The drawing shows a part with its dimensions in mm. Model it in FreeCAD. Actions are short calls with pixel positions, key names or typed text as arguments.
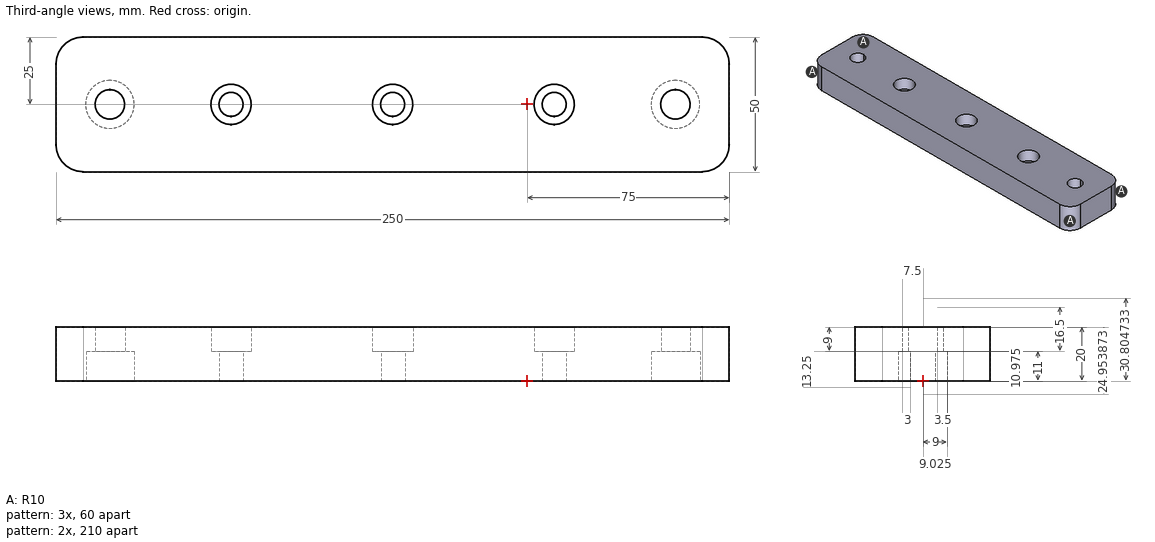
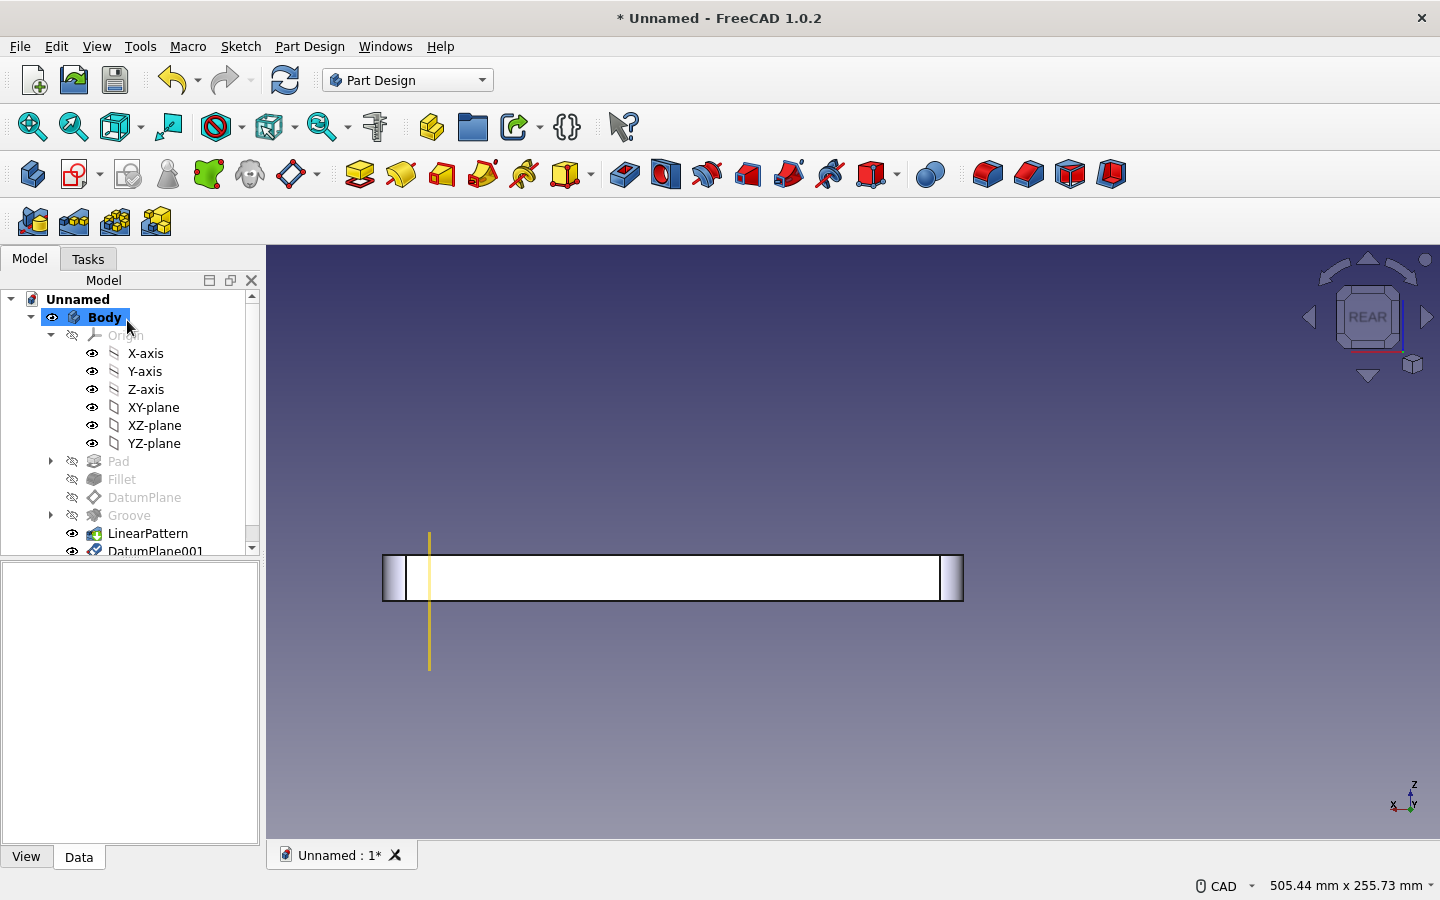
click(117, 551)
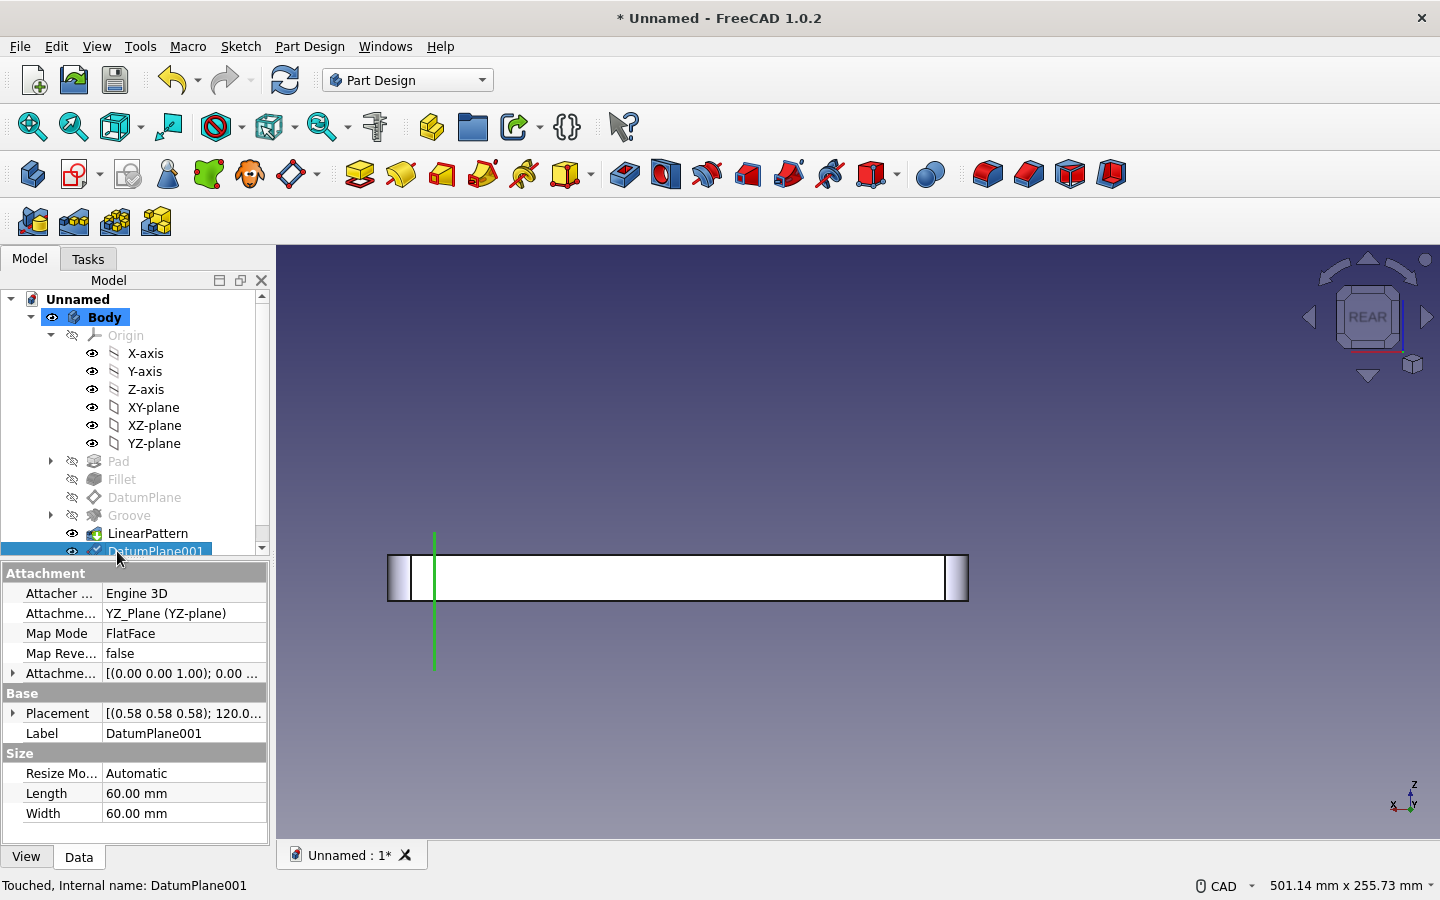
click(74, 174)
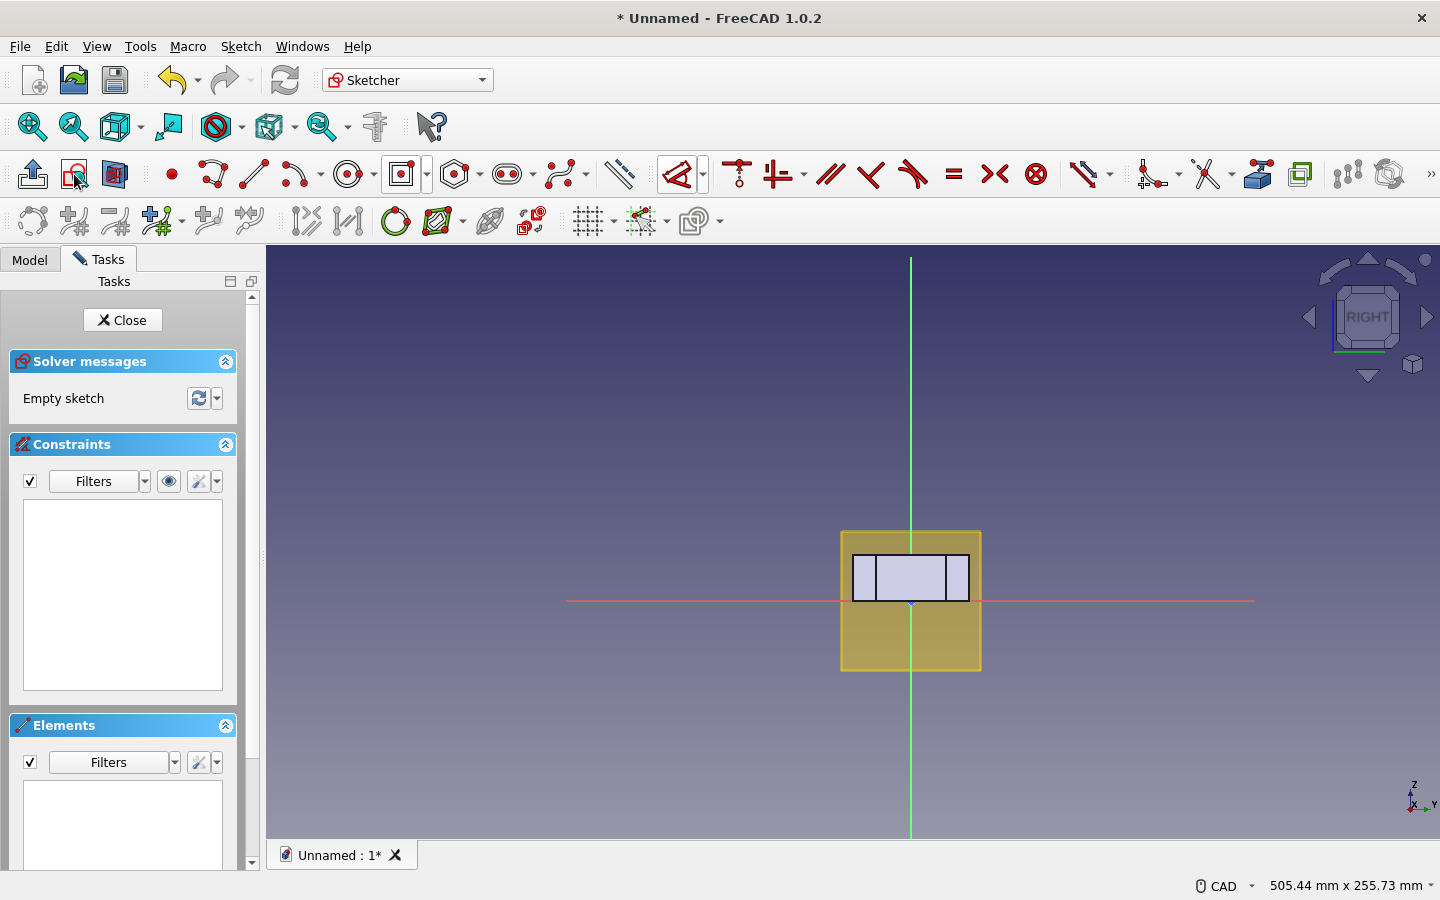
key(q)
key(s)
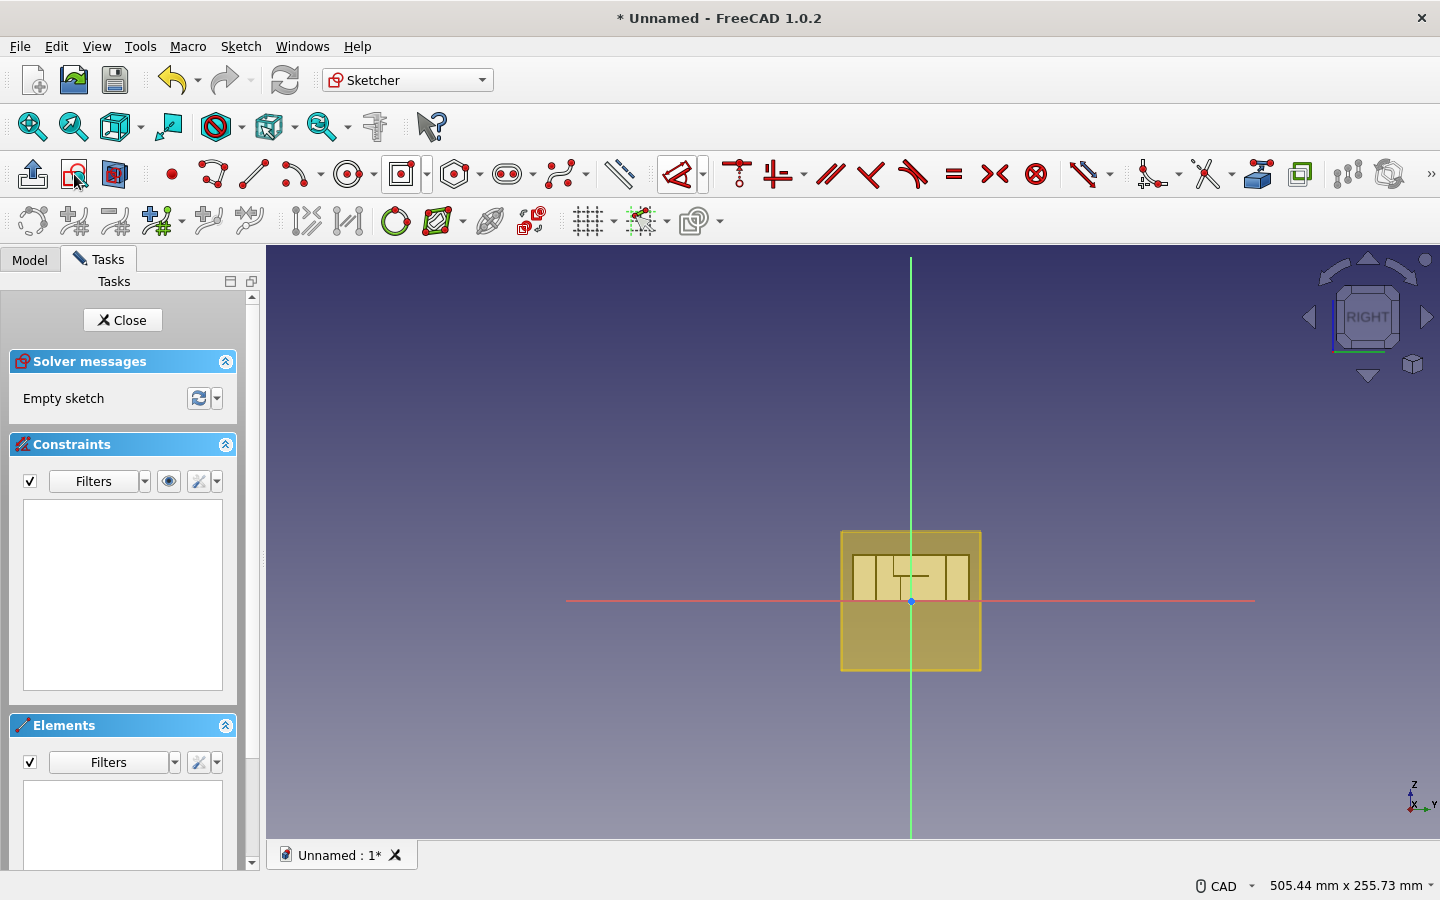
scroll(956, 571, up, 8)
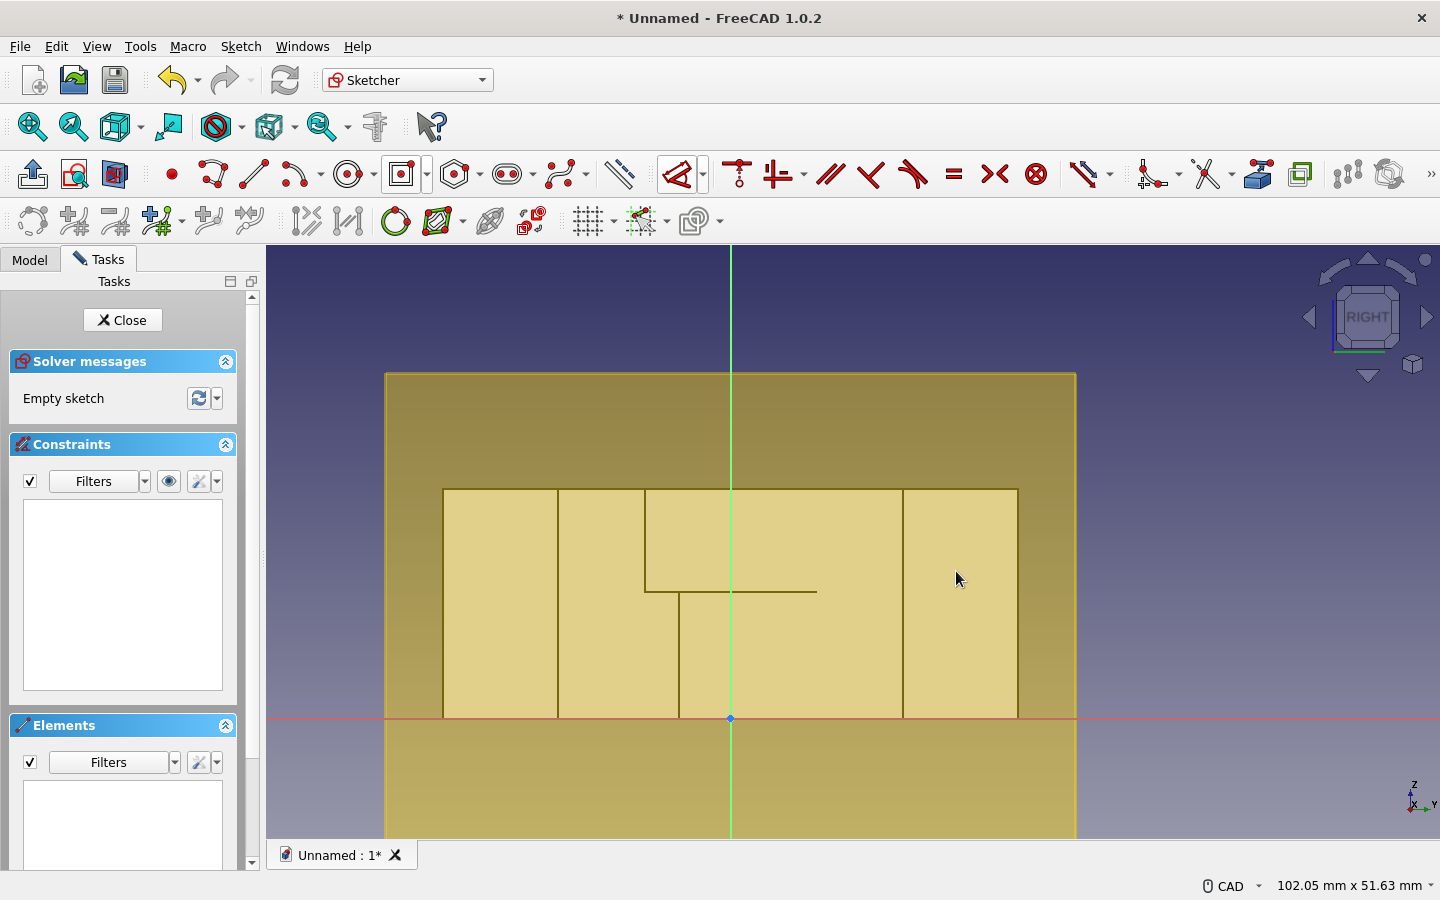
key(g)
key(m)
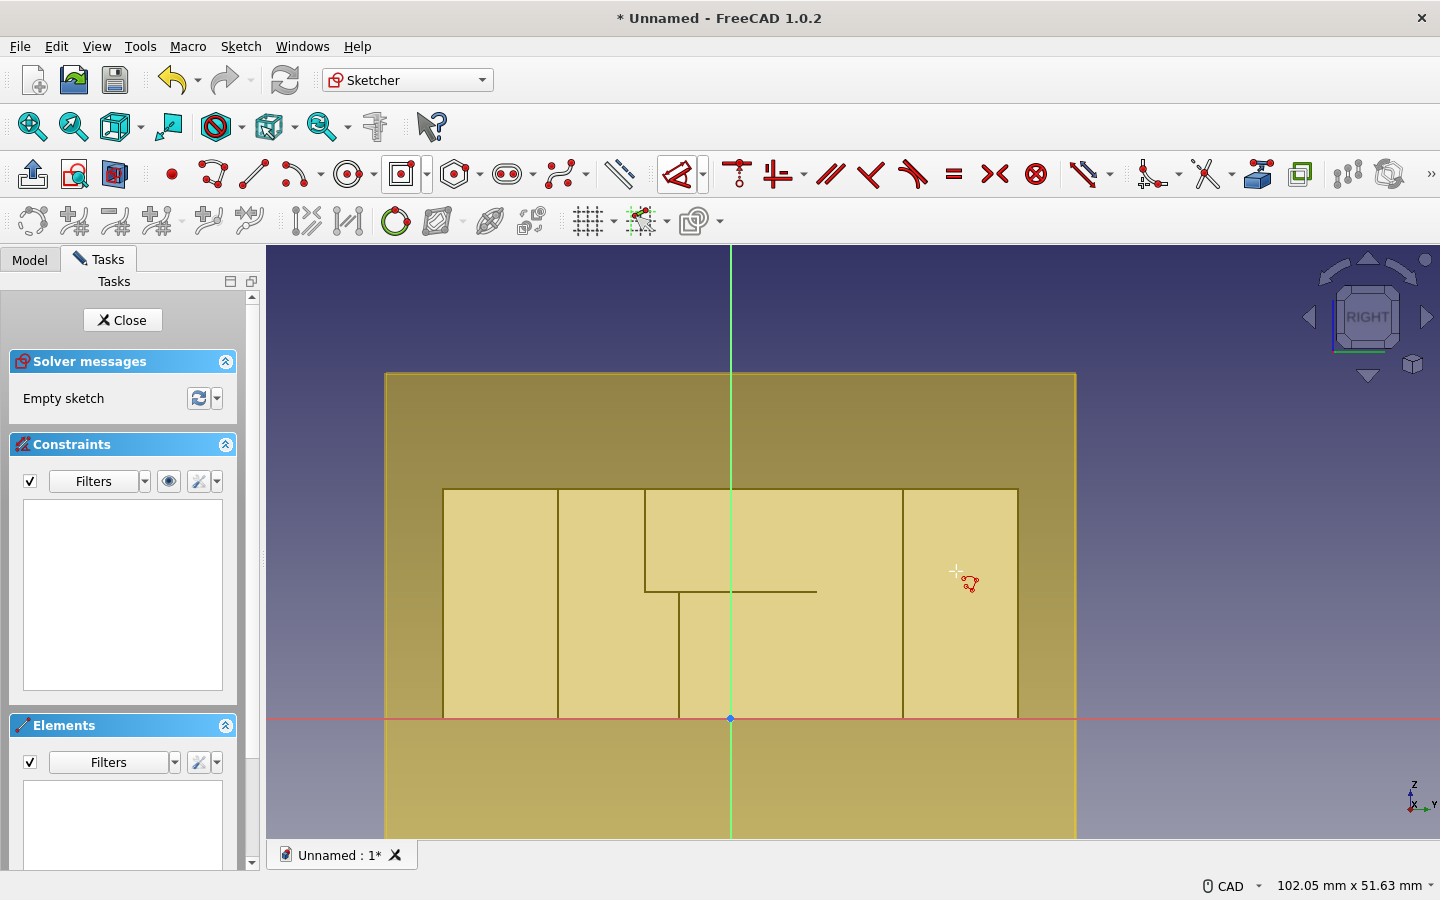
click(731, 719)
click(835, 710)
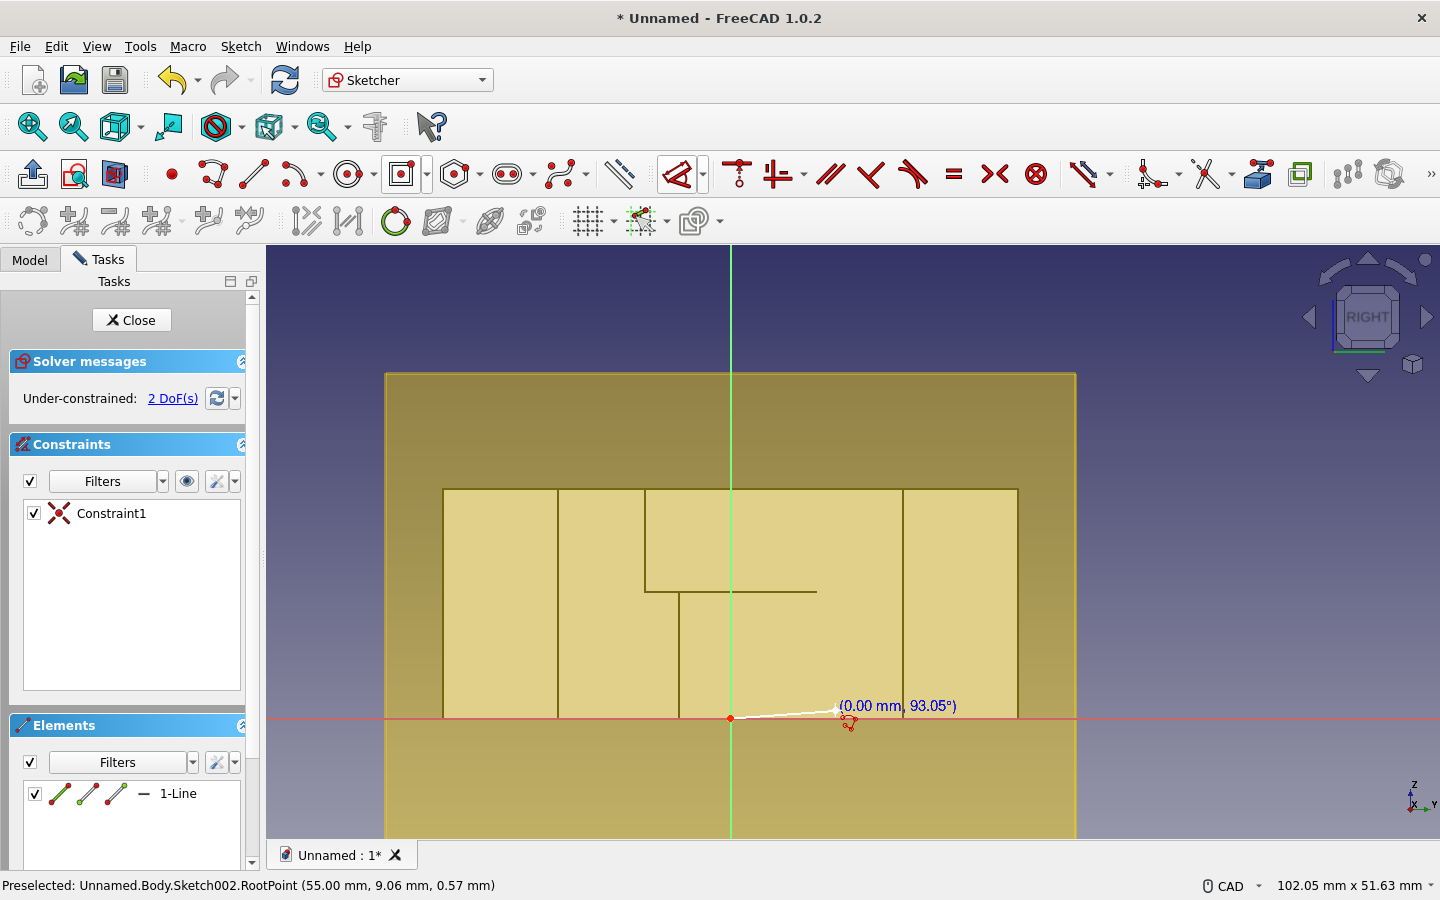
scroll(834, 718, up, 21)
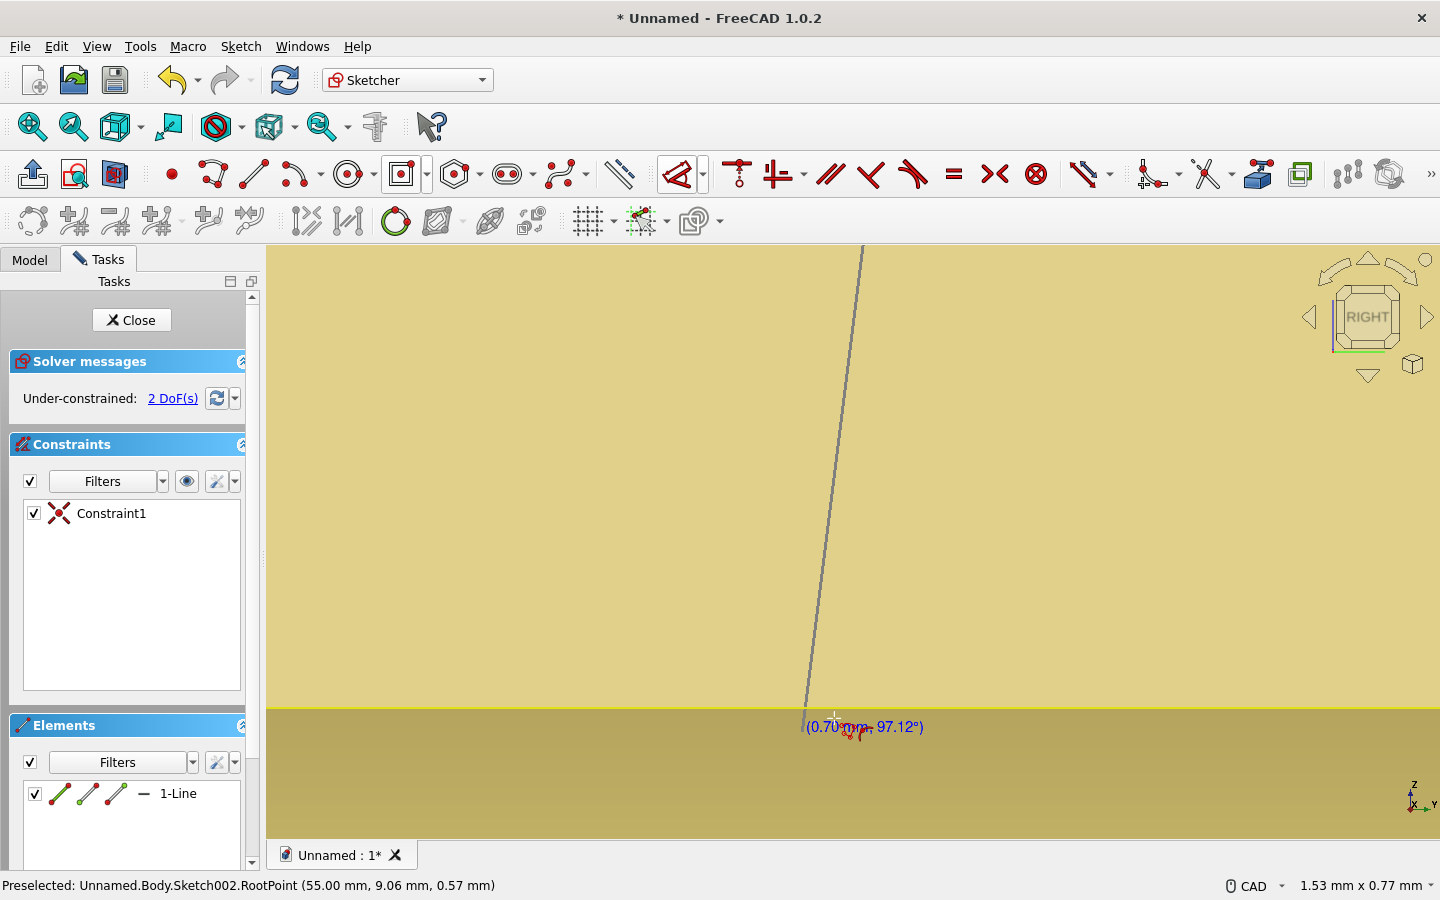
click(829, 689)